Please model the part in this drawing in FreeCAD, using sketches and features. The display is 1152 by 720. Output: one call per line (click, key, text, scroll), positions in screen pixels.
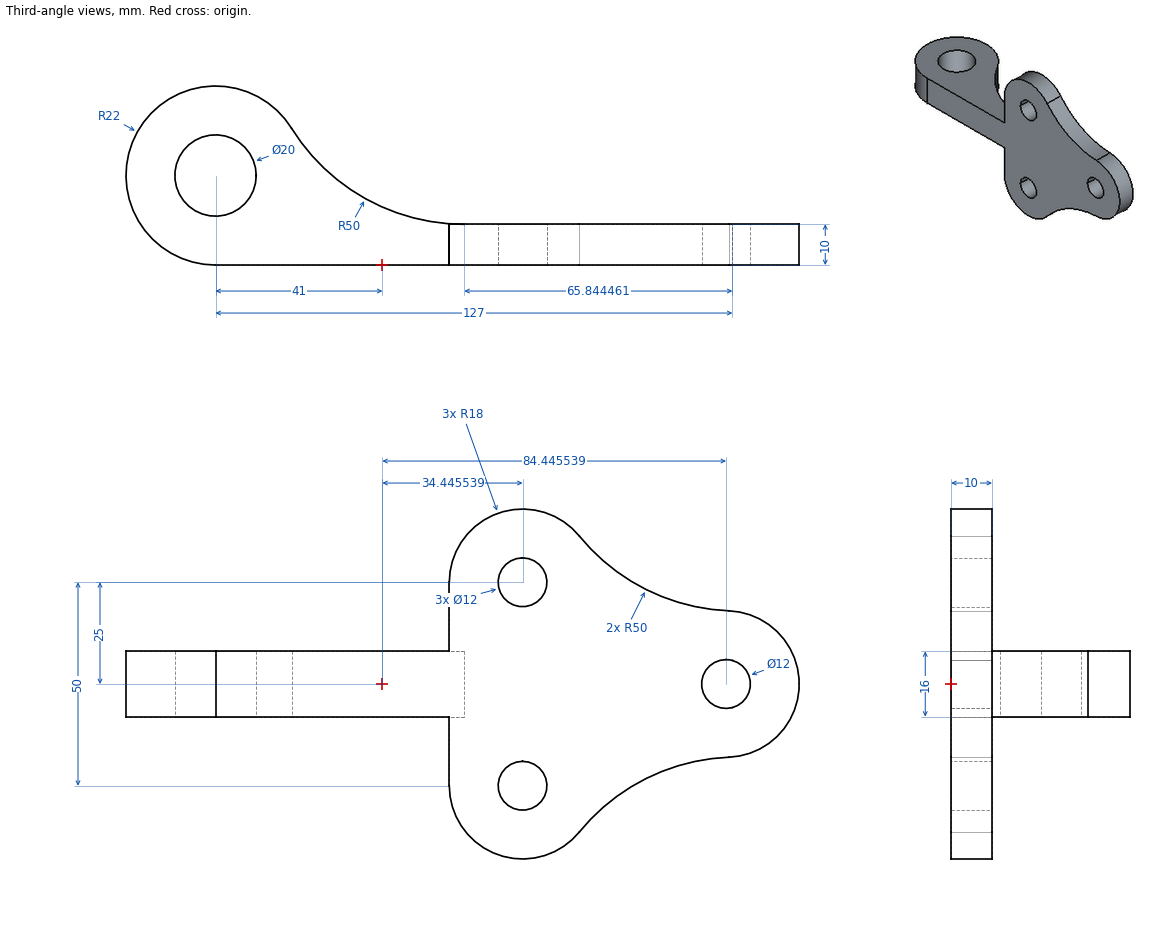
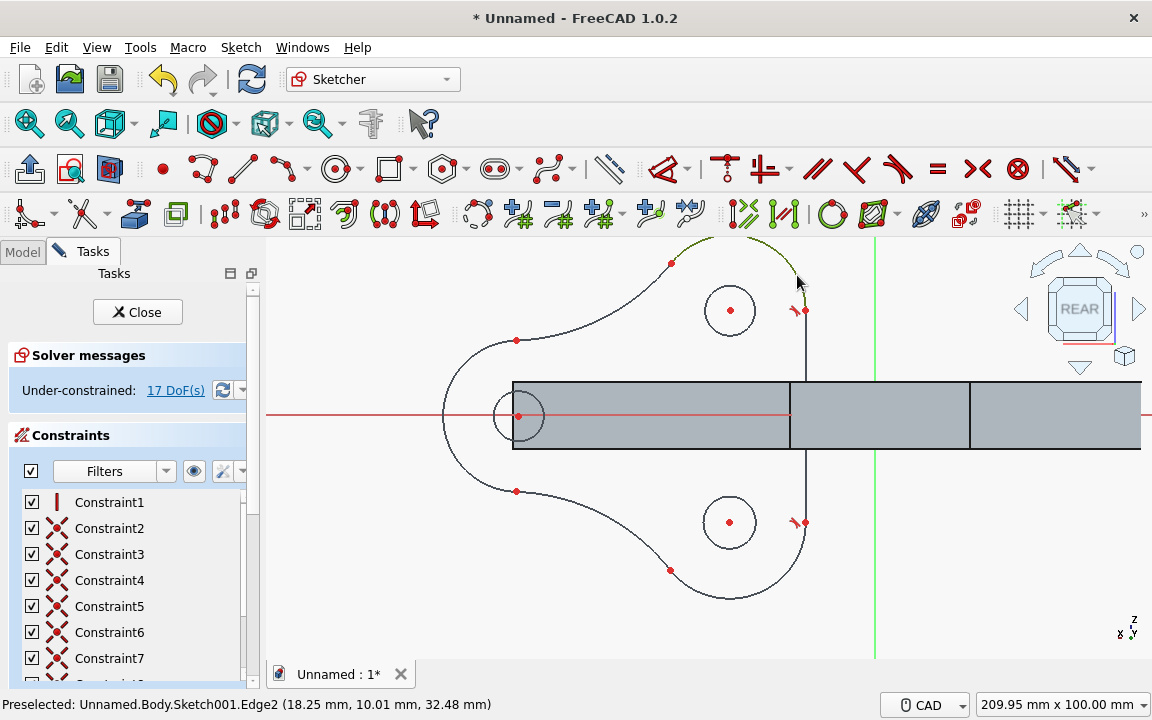
click(569, 332)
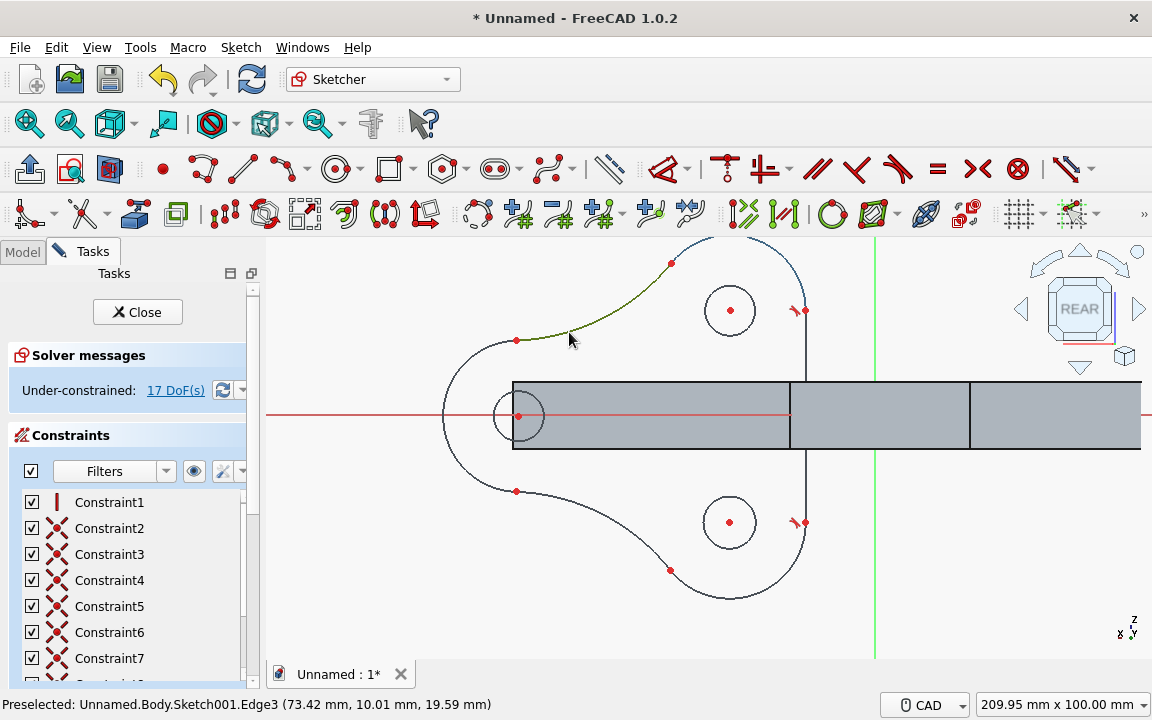
key(t)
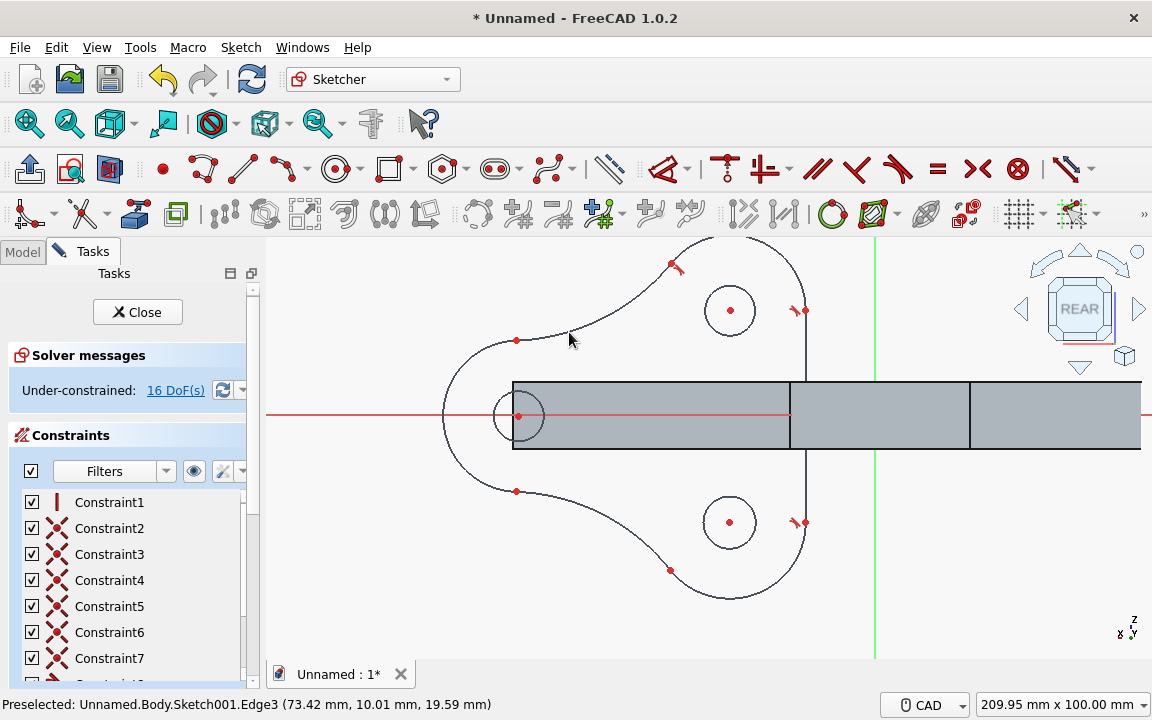
click(569, 332)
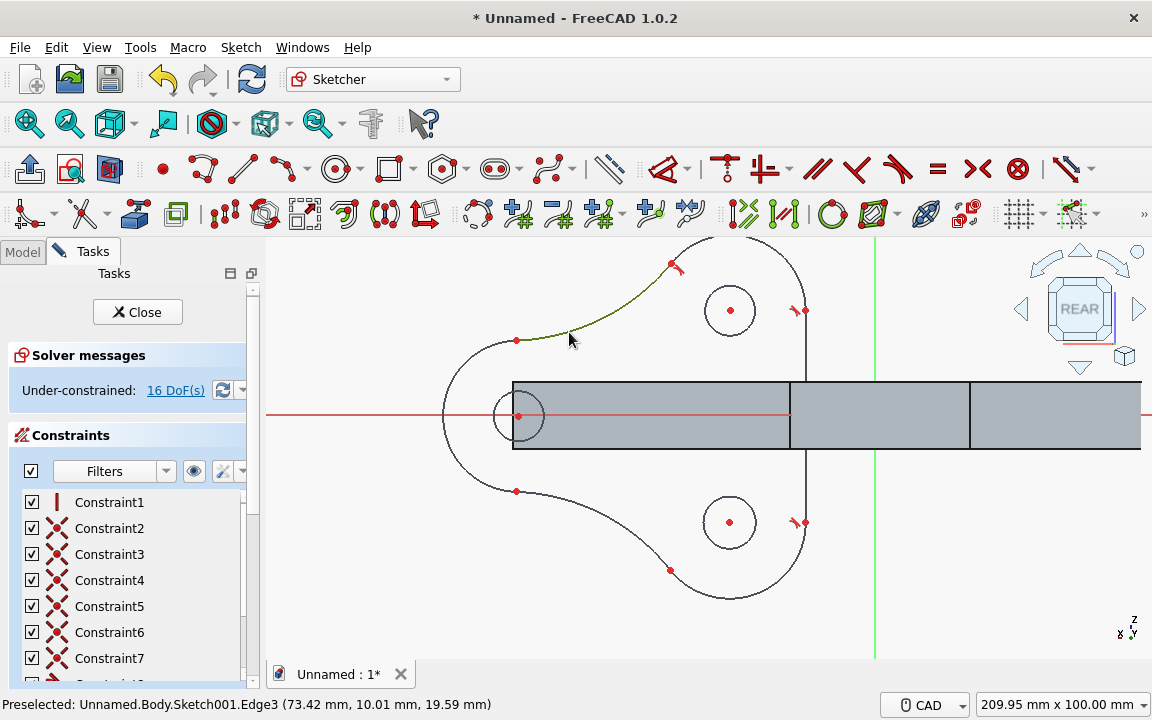
click(457, 373)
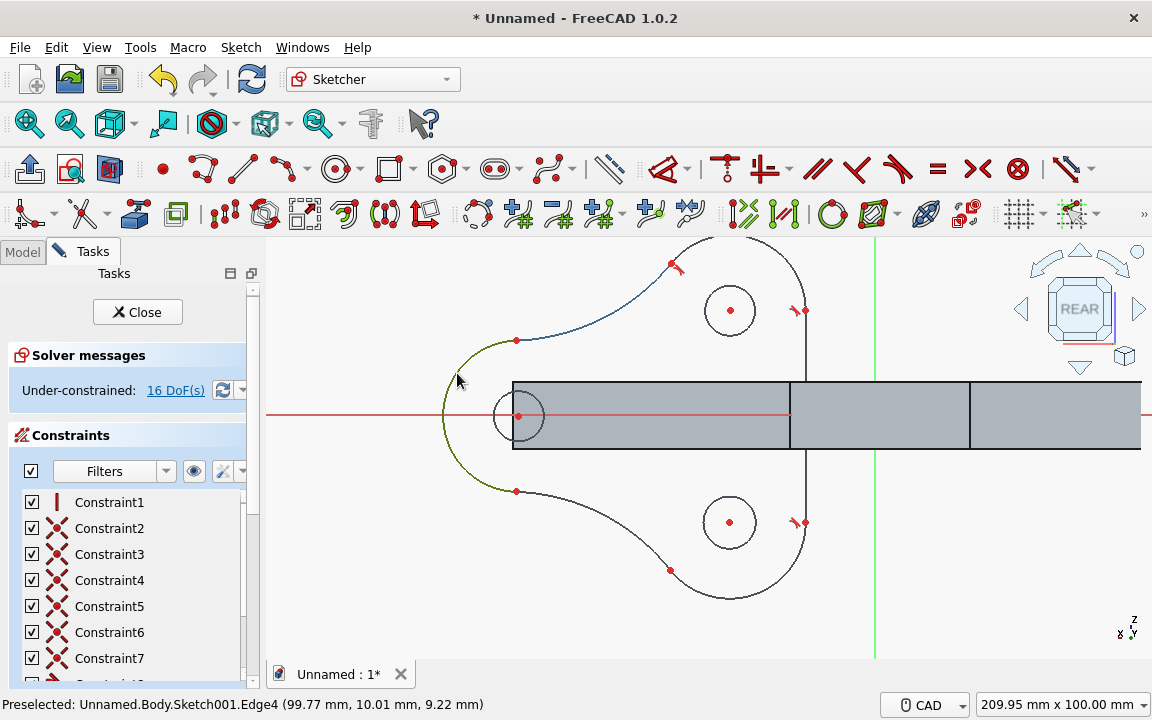
key(t)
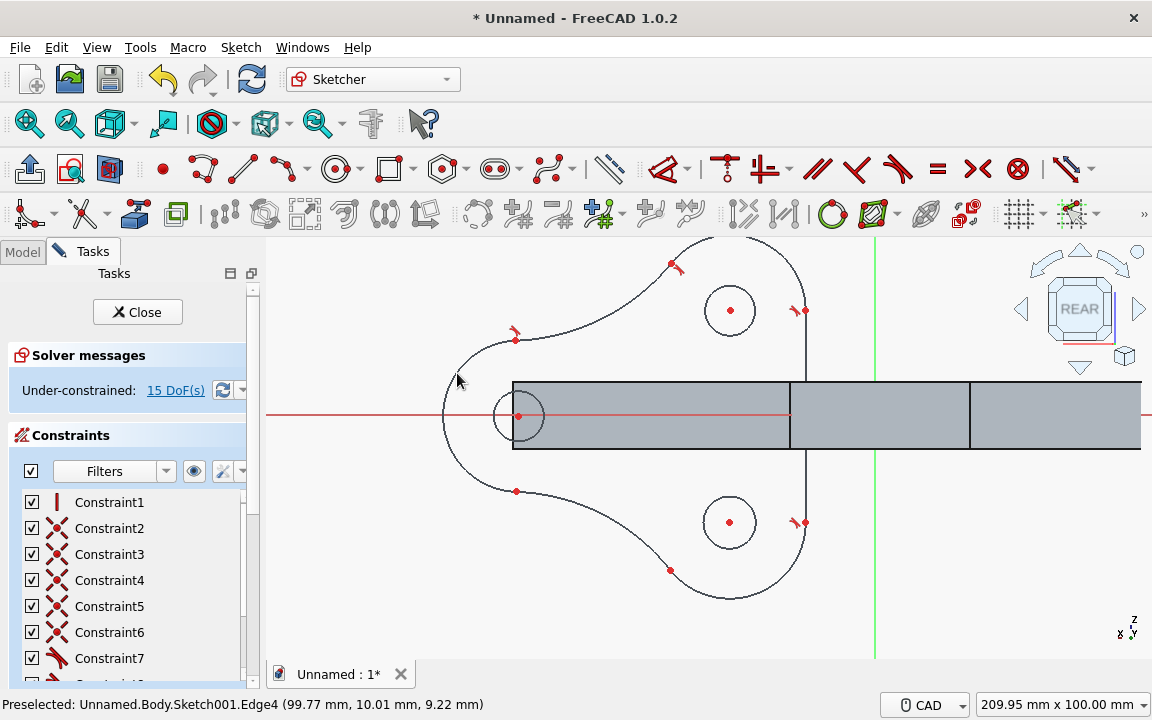
click(457, 373)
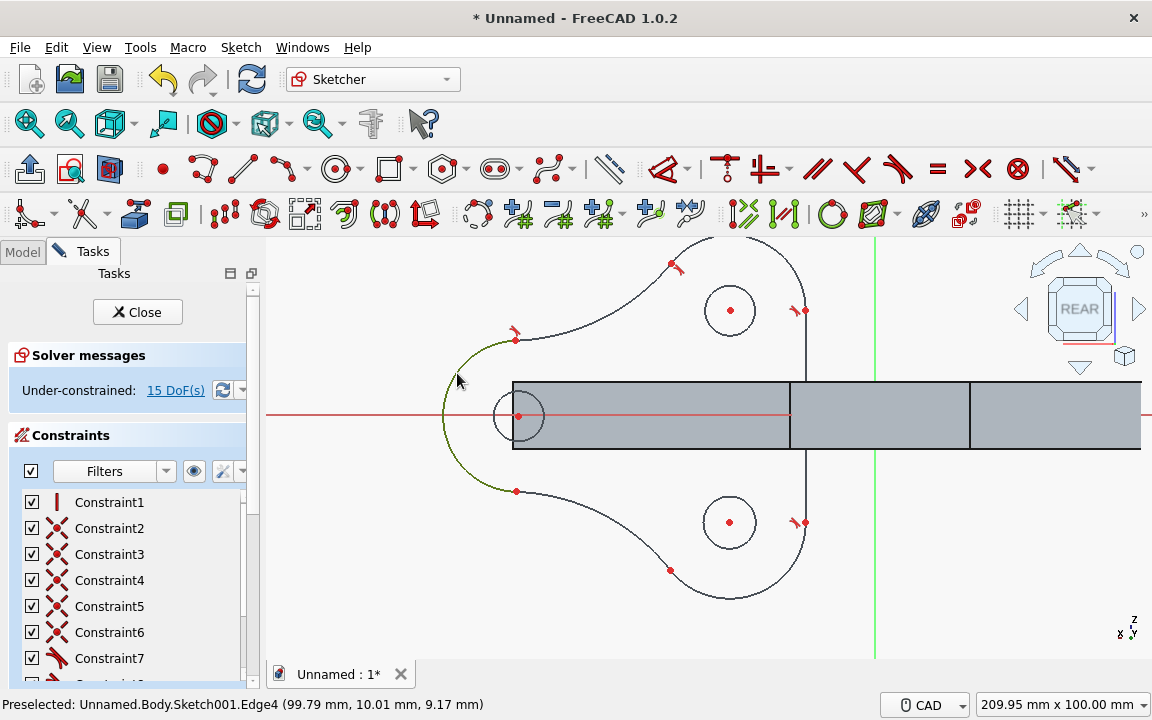
click(632, 533)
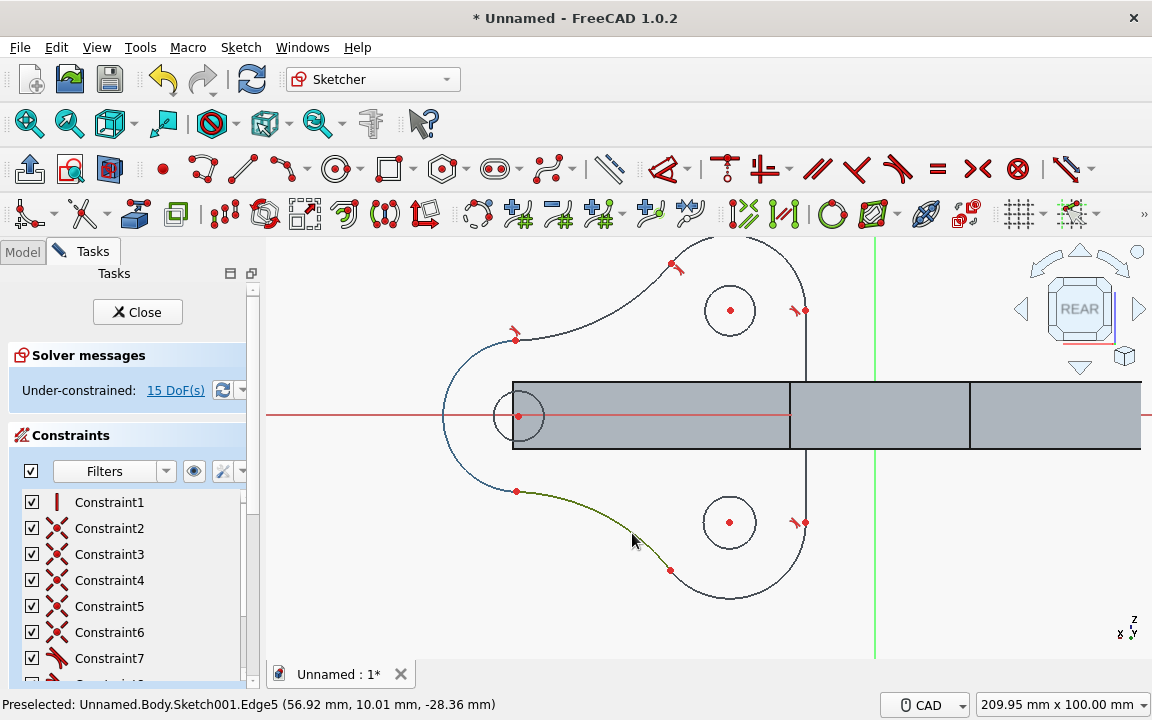
key(t)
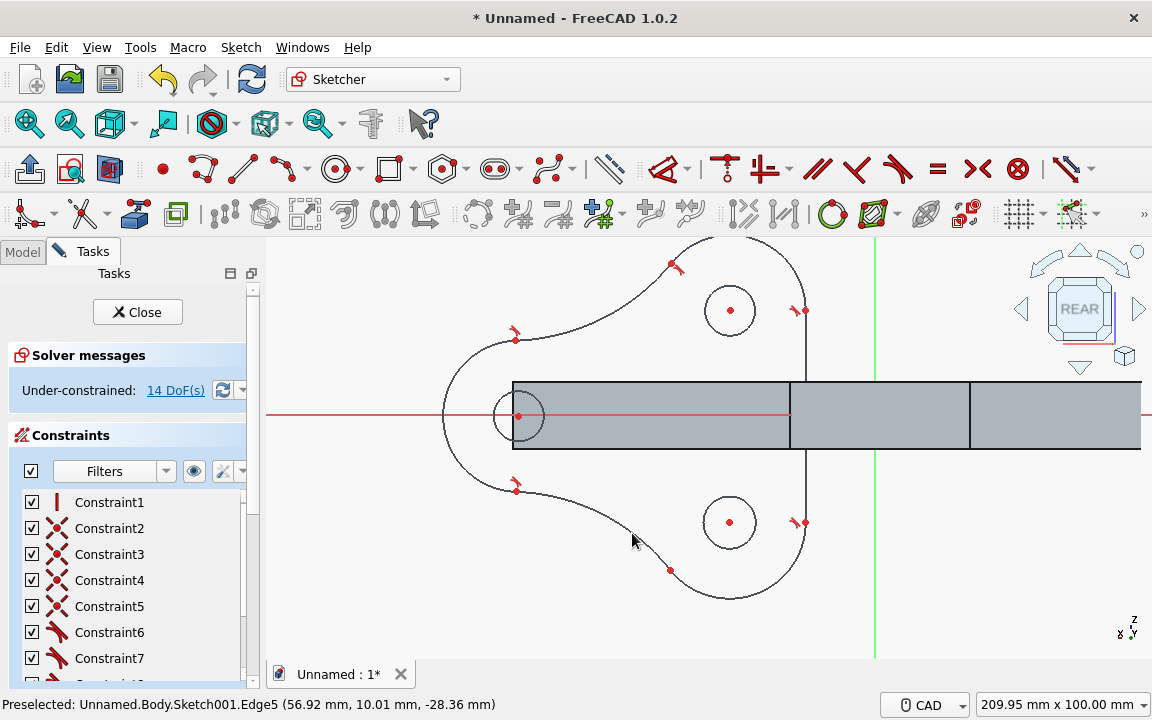
click(632, 533)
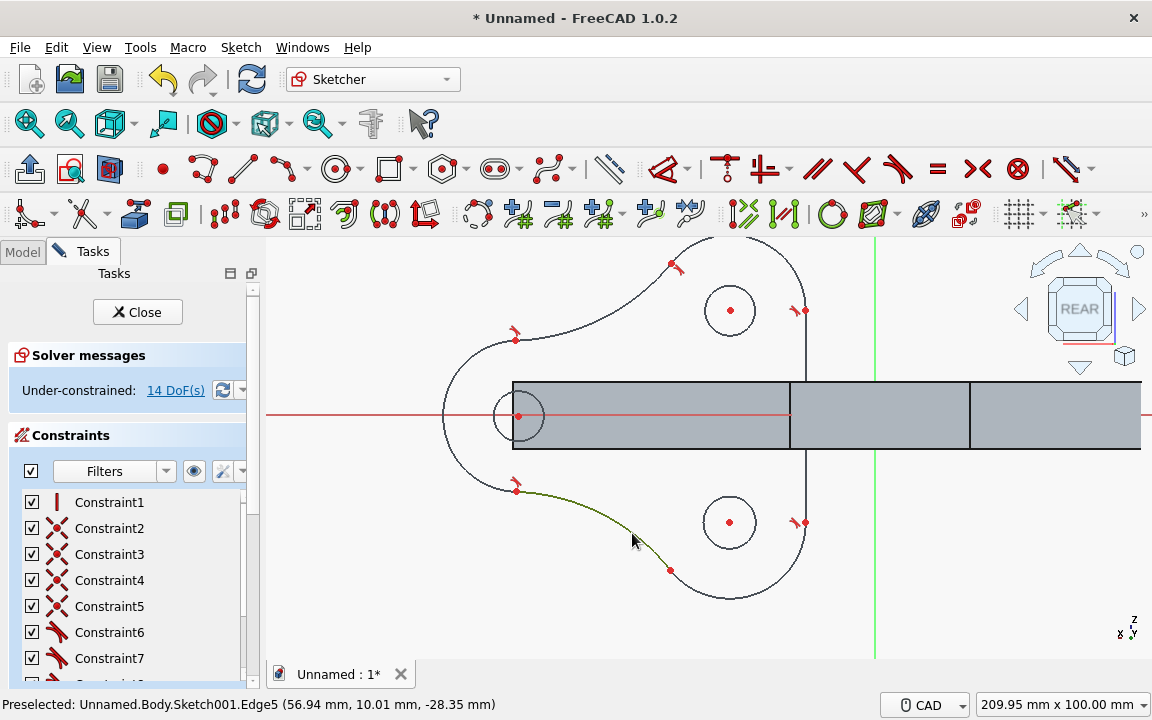
click(718, 598)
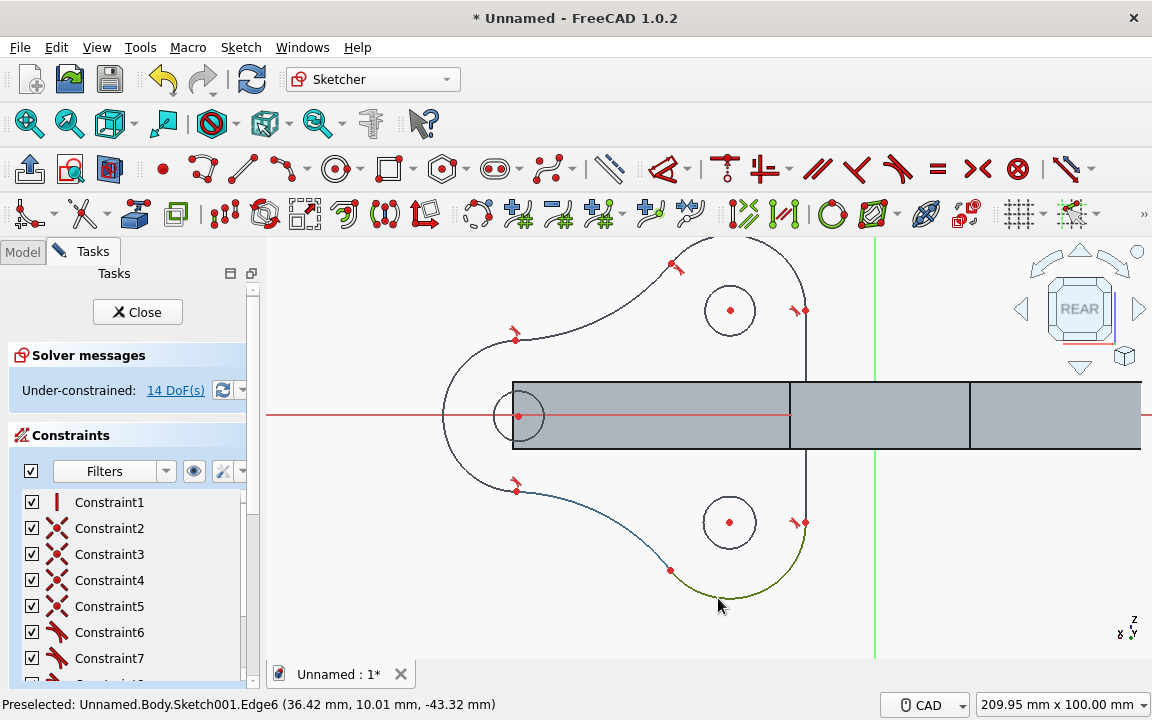
key(t)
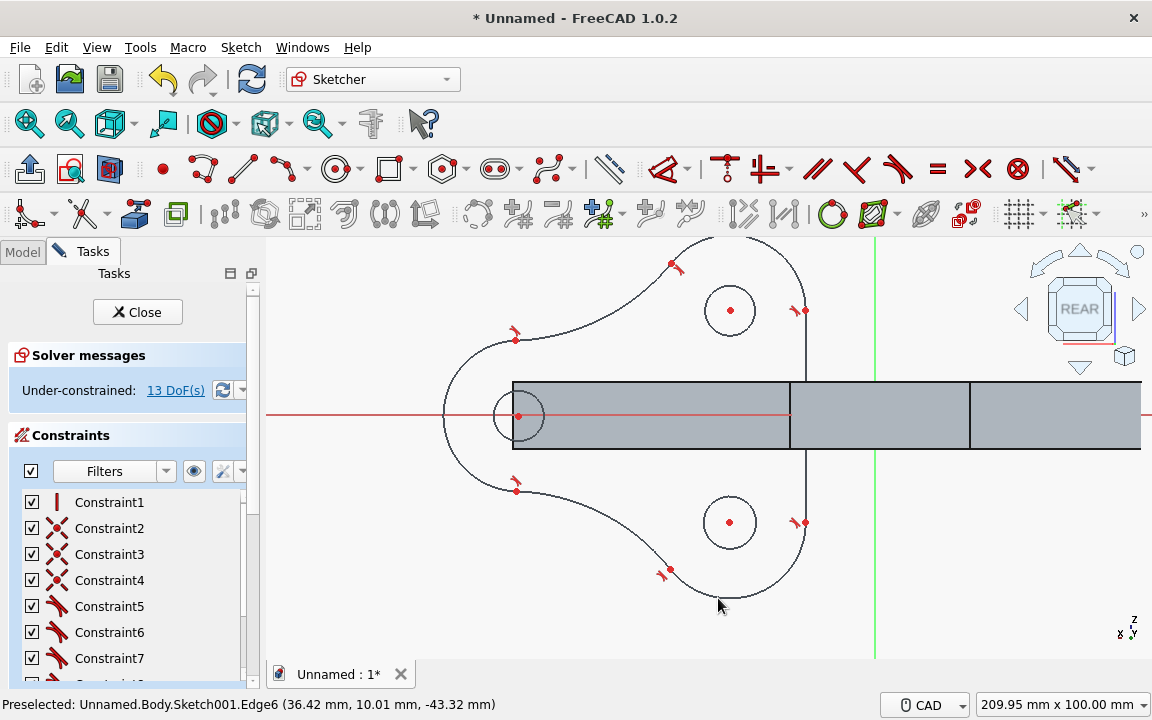
click(797, 275)